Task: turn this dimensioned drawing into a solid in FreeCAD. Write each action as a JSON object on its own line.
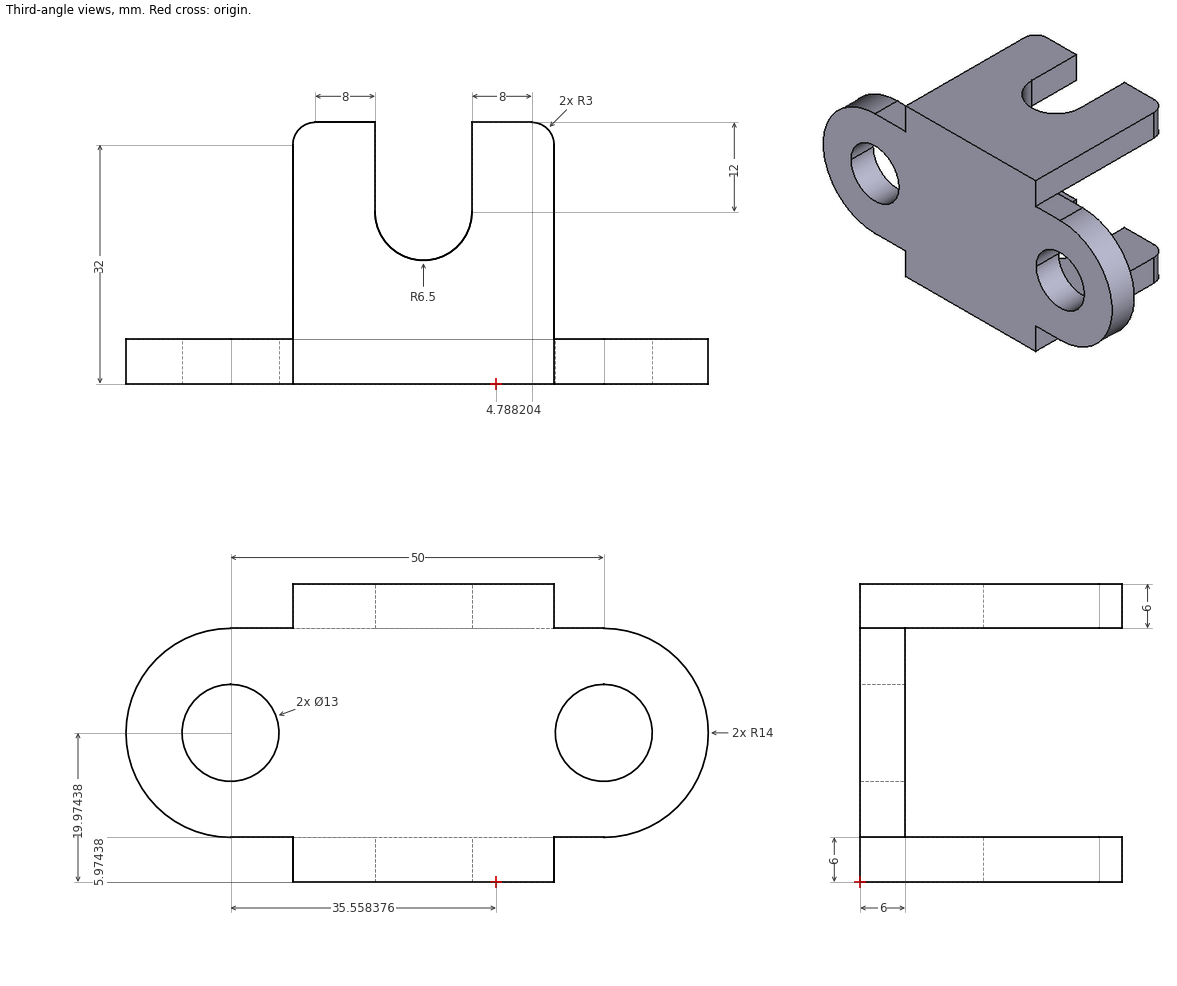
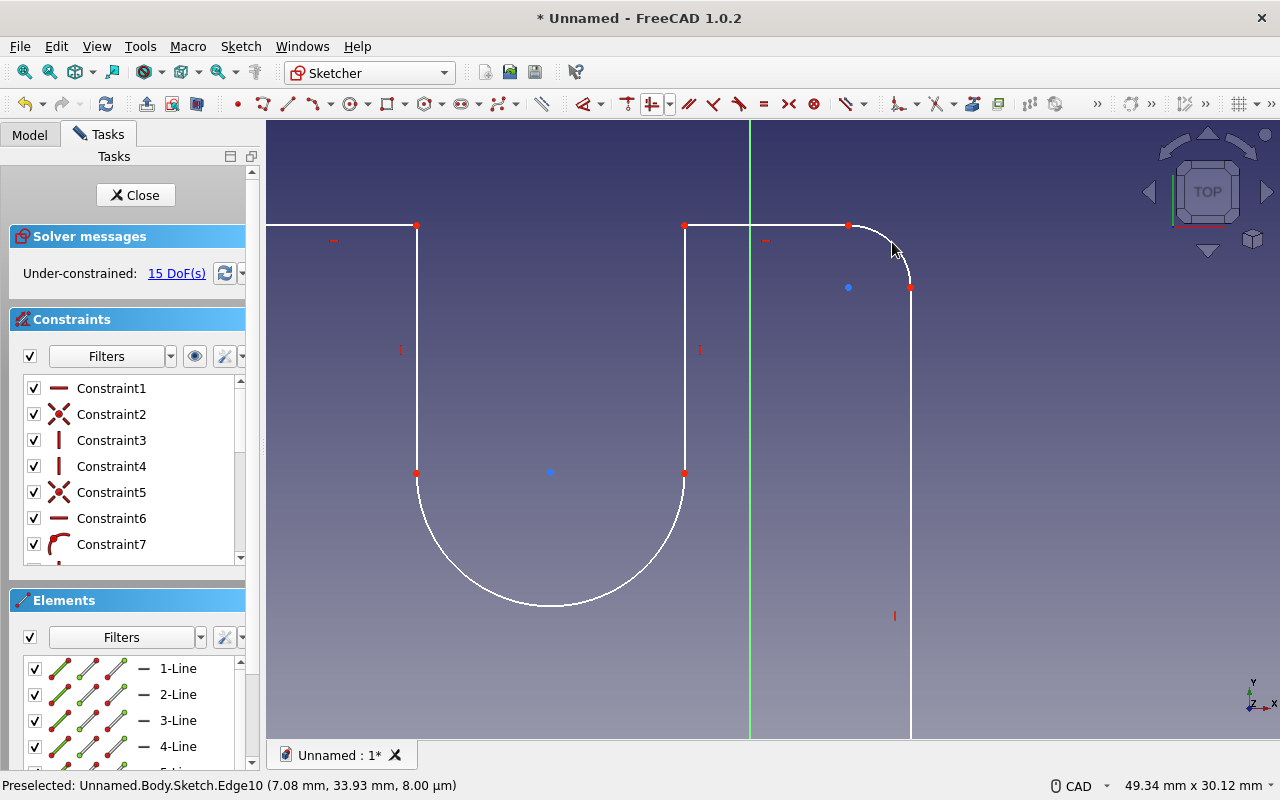
{"action": "left_click", "coordinate": [799, 225]}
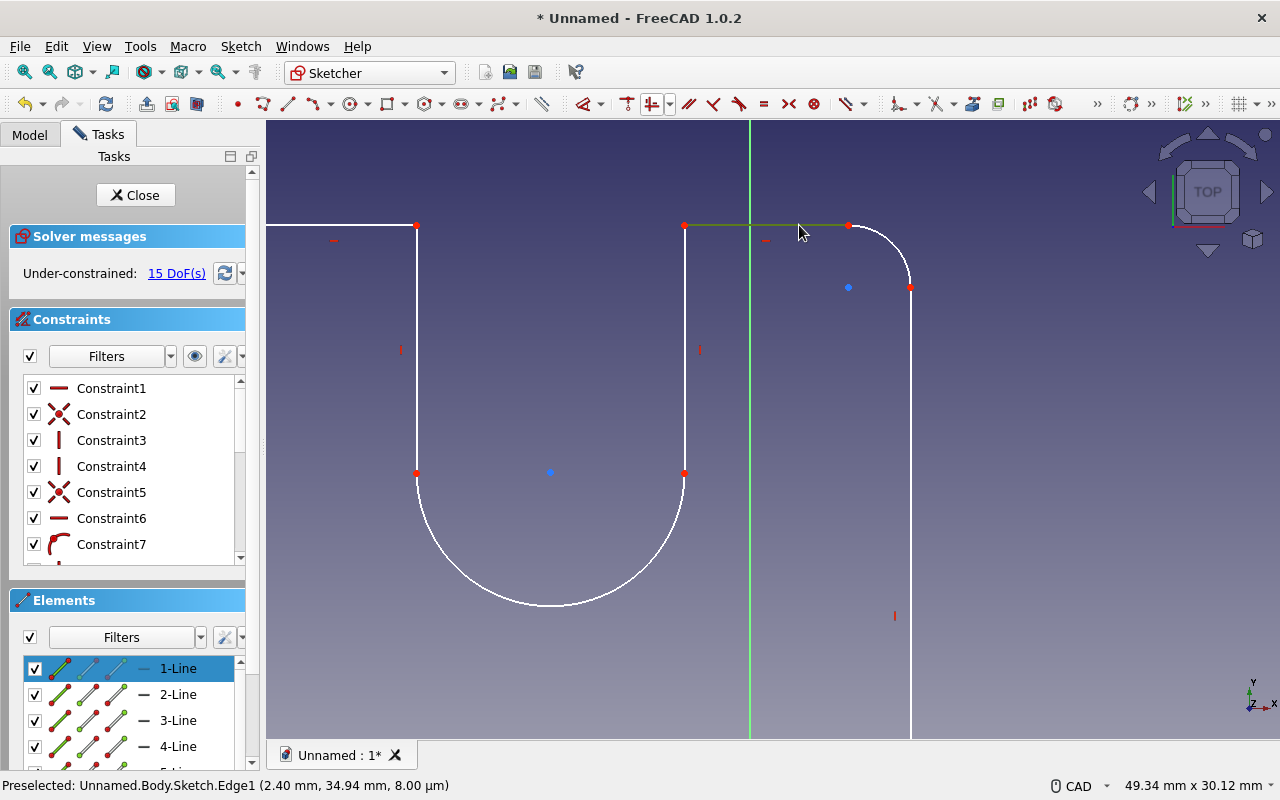
{"action": "left_click", "coordinate": [904, 259]}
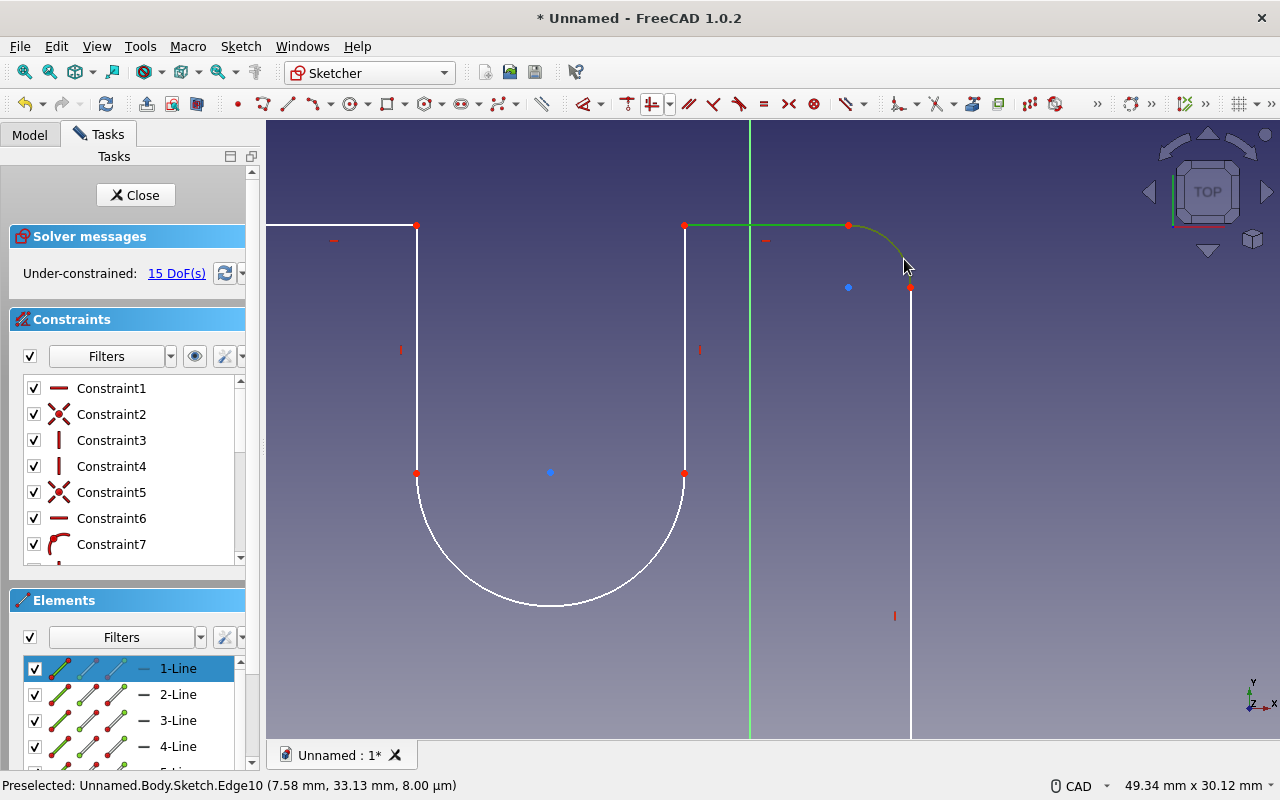
{"action": "left_click", "coordinate": [739, 104]}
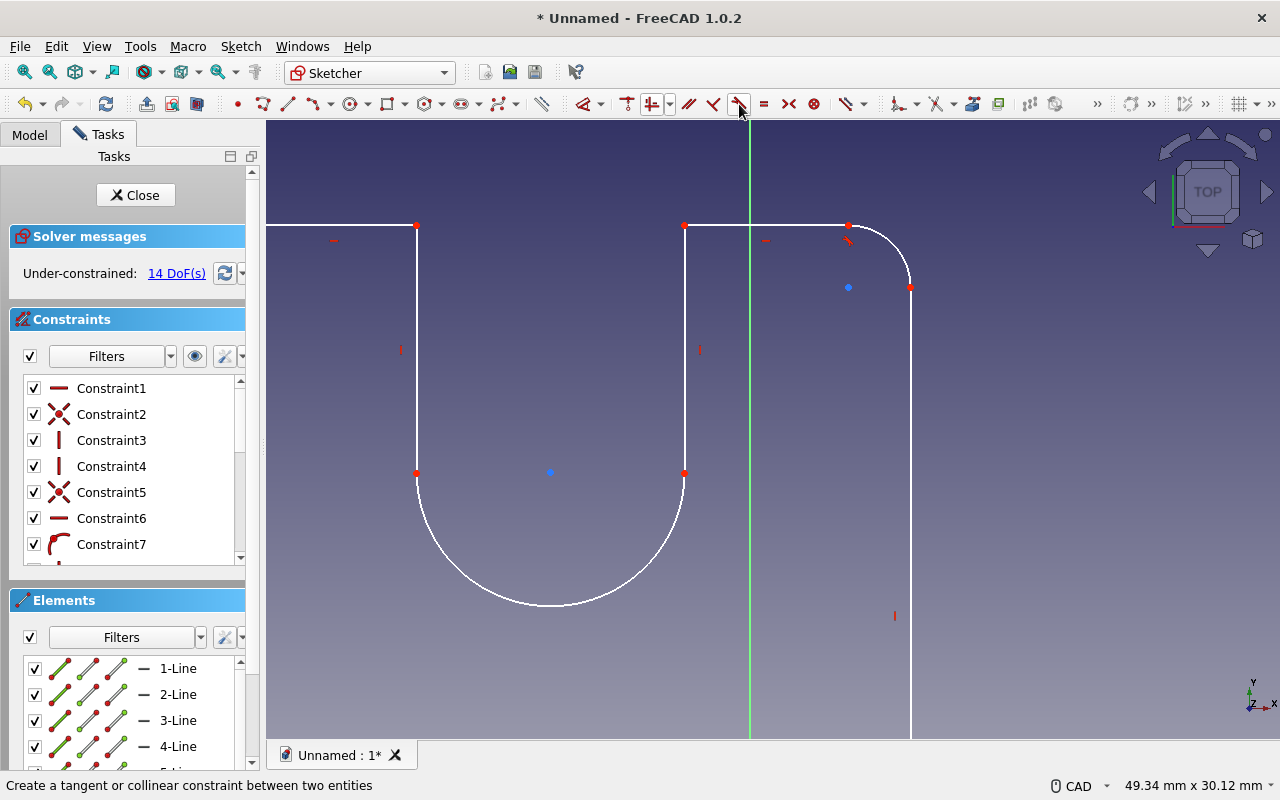
{"action": "left_click", "coordinate": [685, 300]}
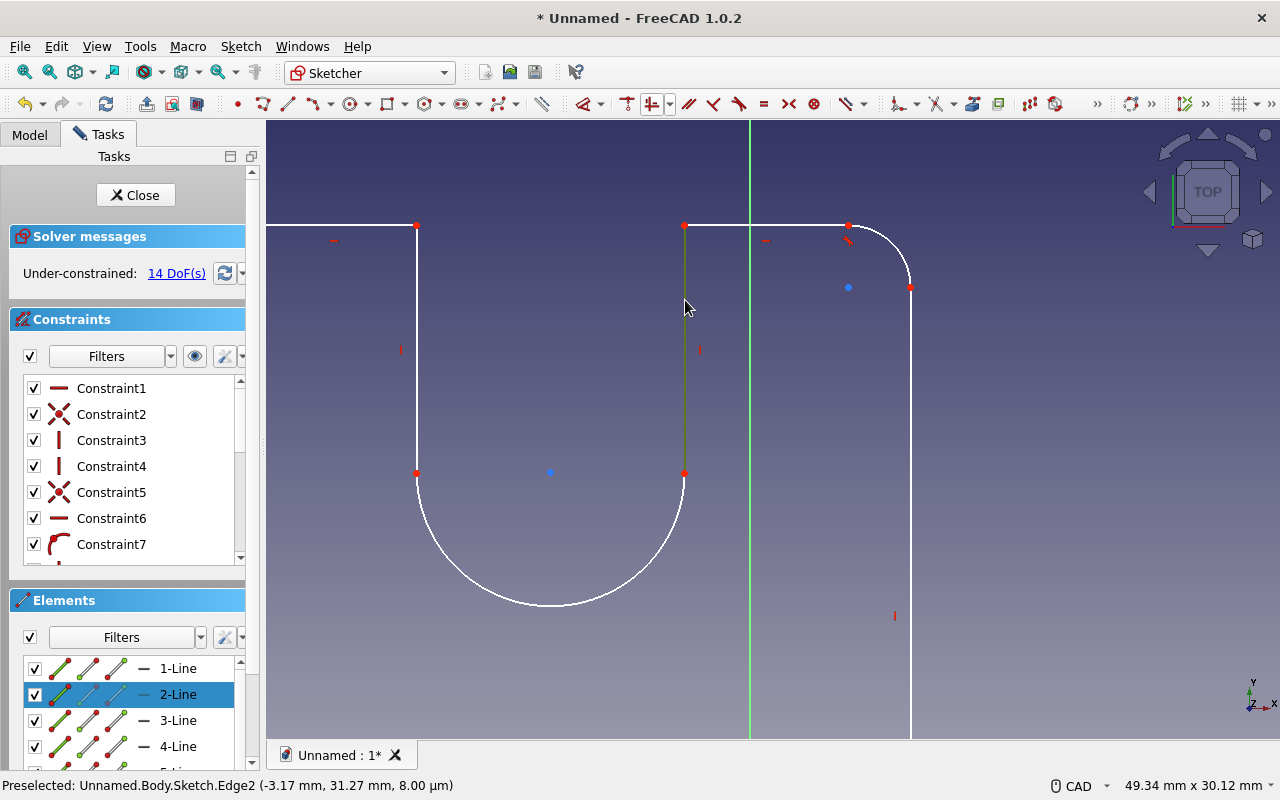
{"action": "left_click", "coordinate": [472, 581]}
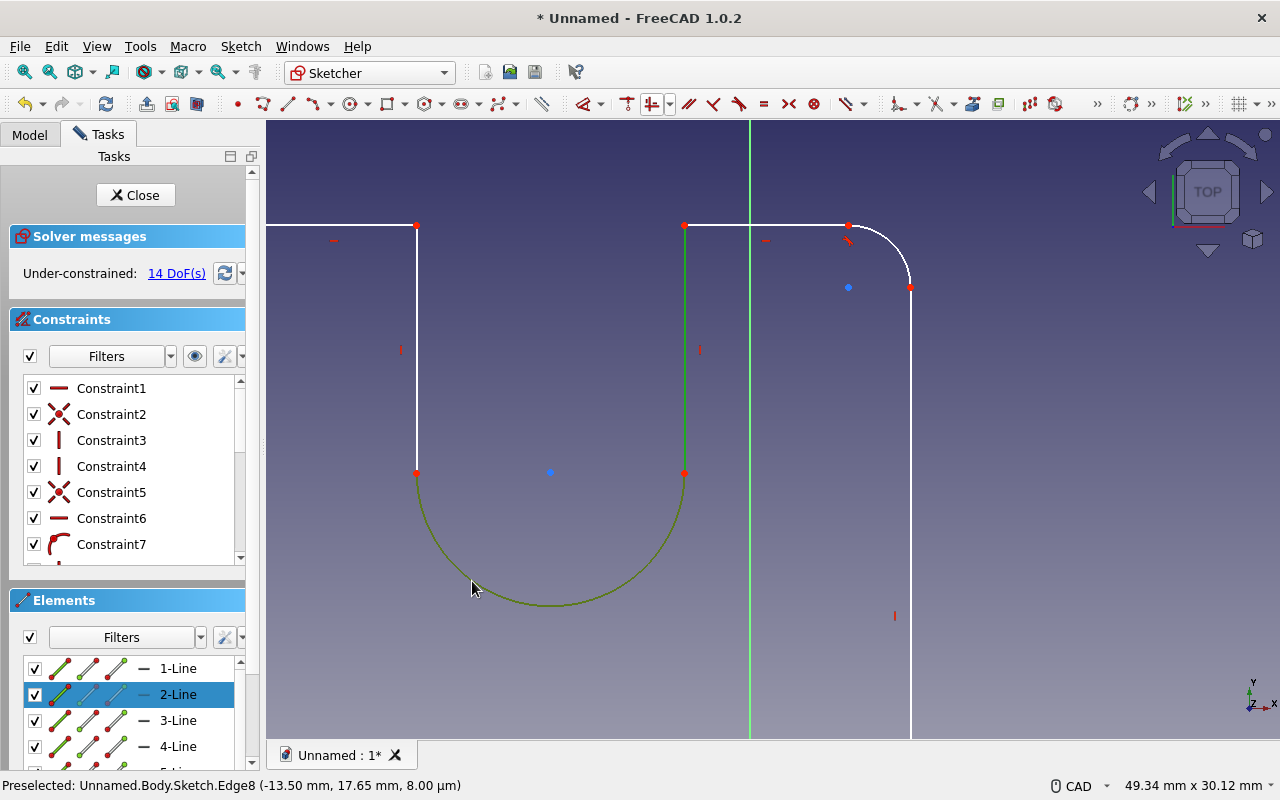
{"action": "left_click", "coordinate": [739, 104]}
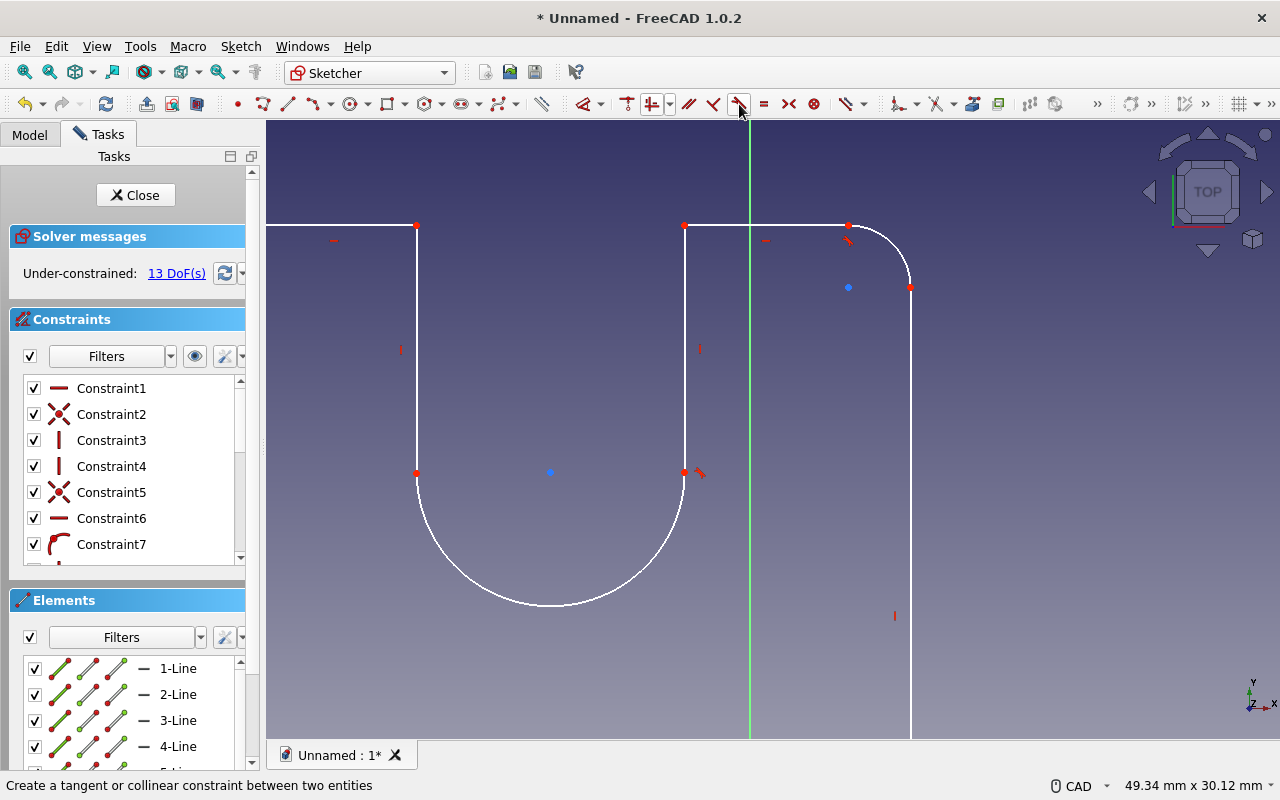
{"action": "left_click", "coordinate": [417, 399]}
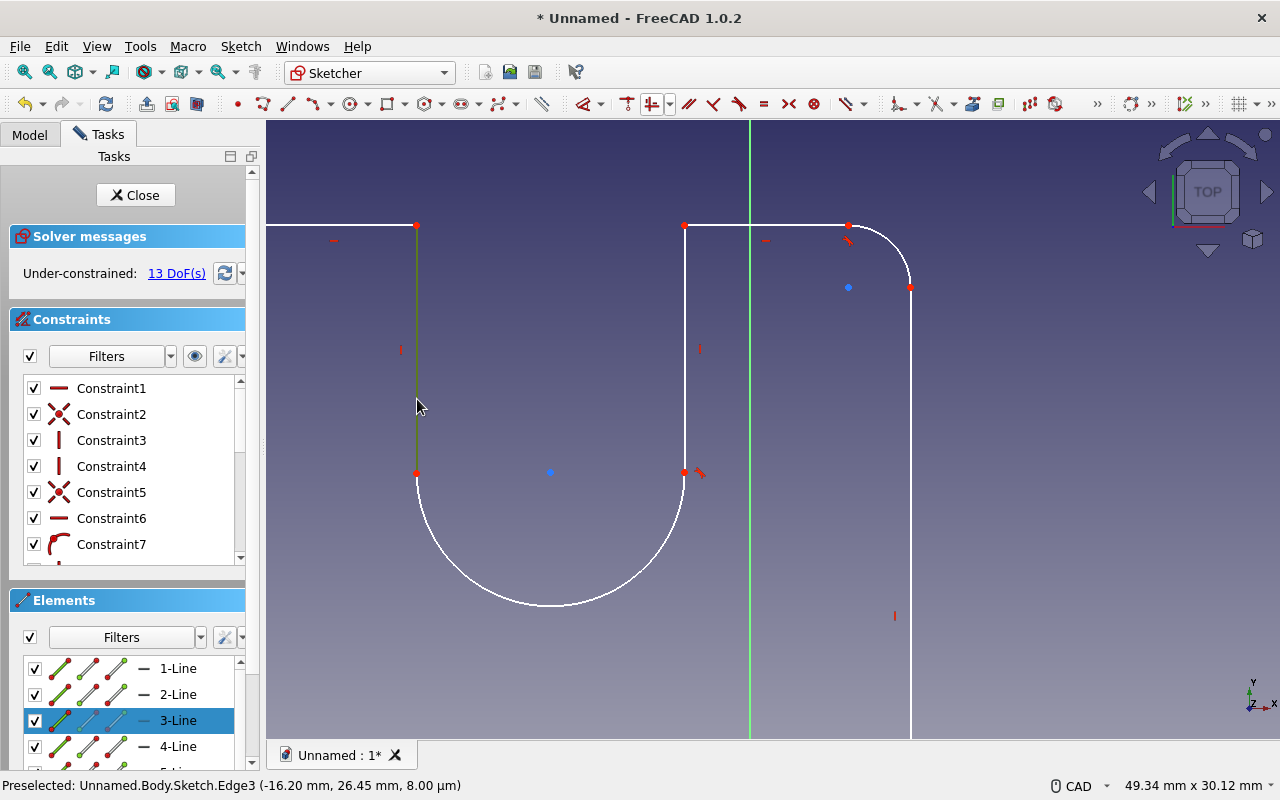
{"action": "left_click", "coordinate": [472, 581]}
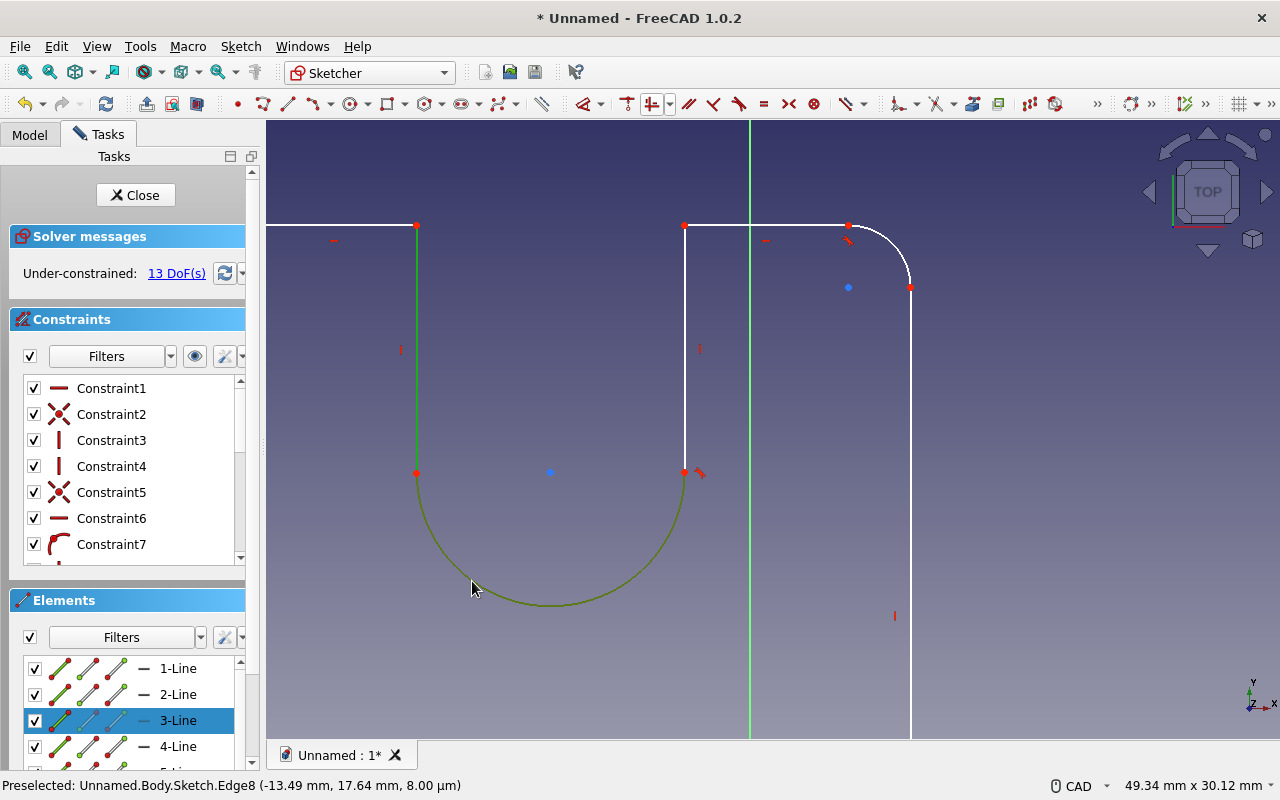
{"action": "left_click", "coordinate": [739, 104]}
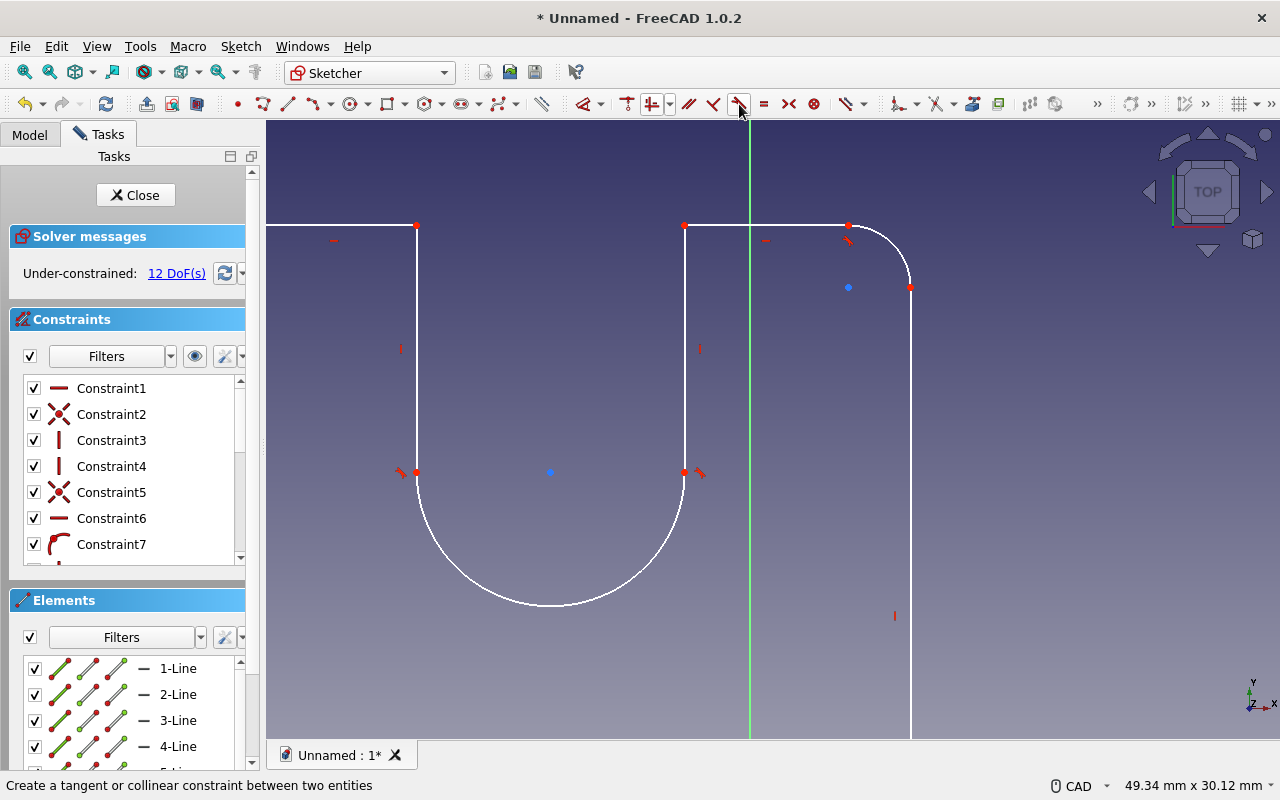
{"action": "left_click", "coordinate": [368, 225]}